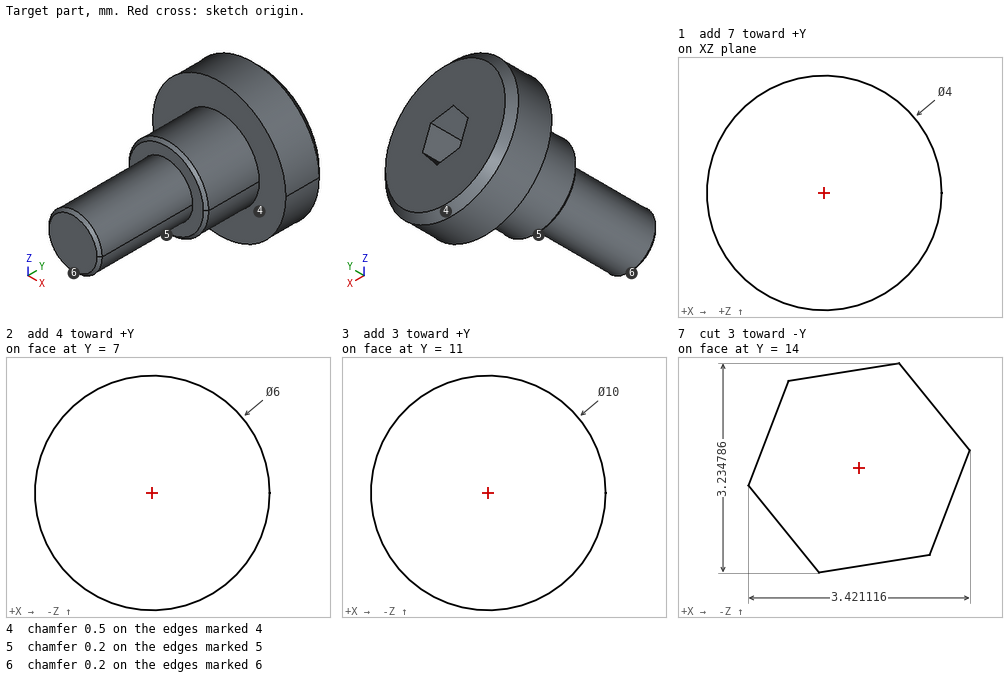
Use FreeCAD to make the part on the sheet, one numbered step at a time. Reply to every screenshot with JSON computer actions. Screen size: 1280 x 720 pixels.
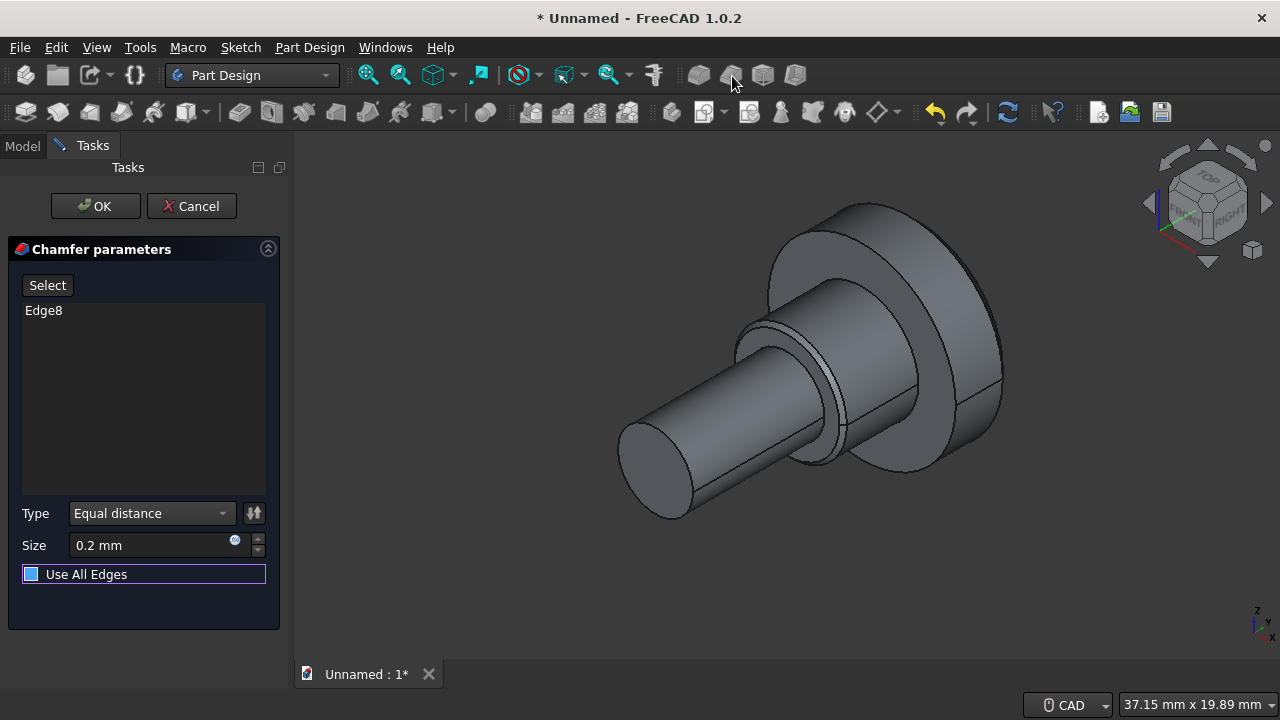
{"action": "left_click", "coordinate": [96, 206]}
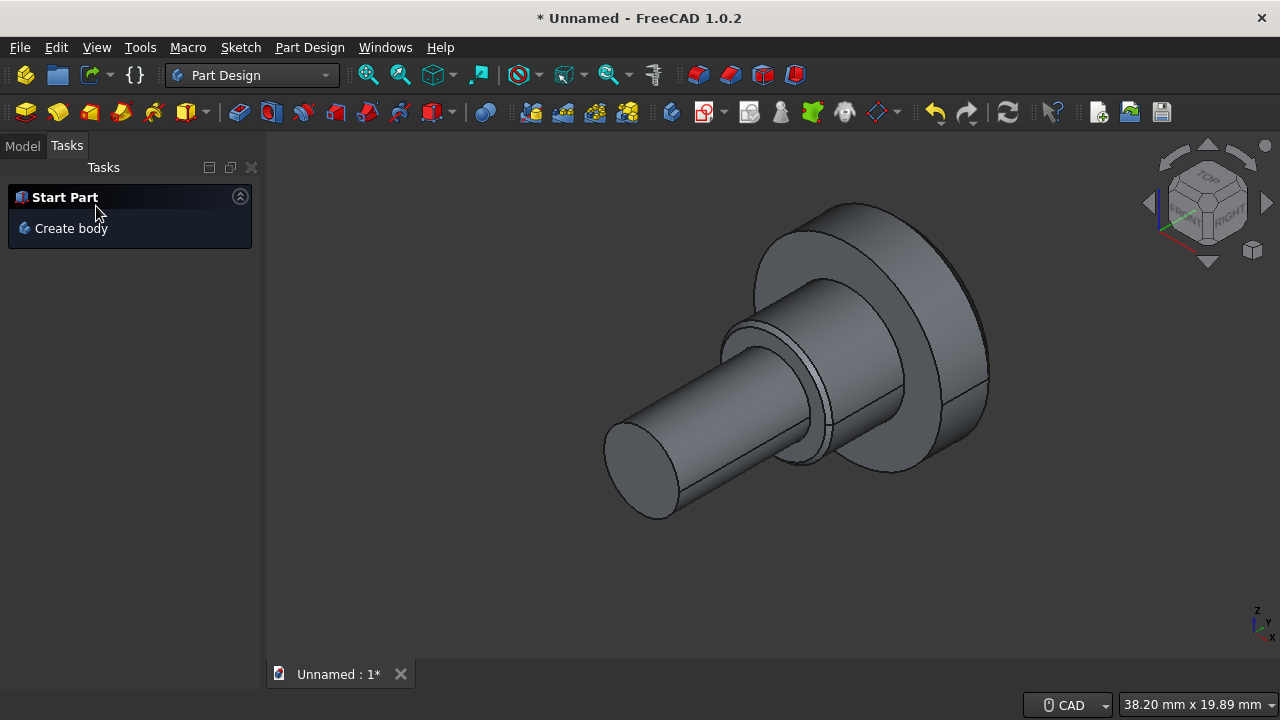
{"action": "left_click", "coordinate": [630, 422]}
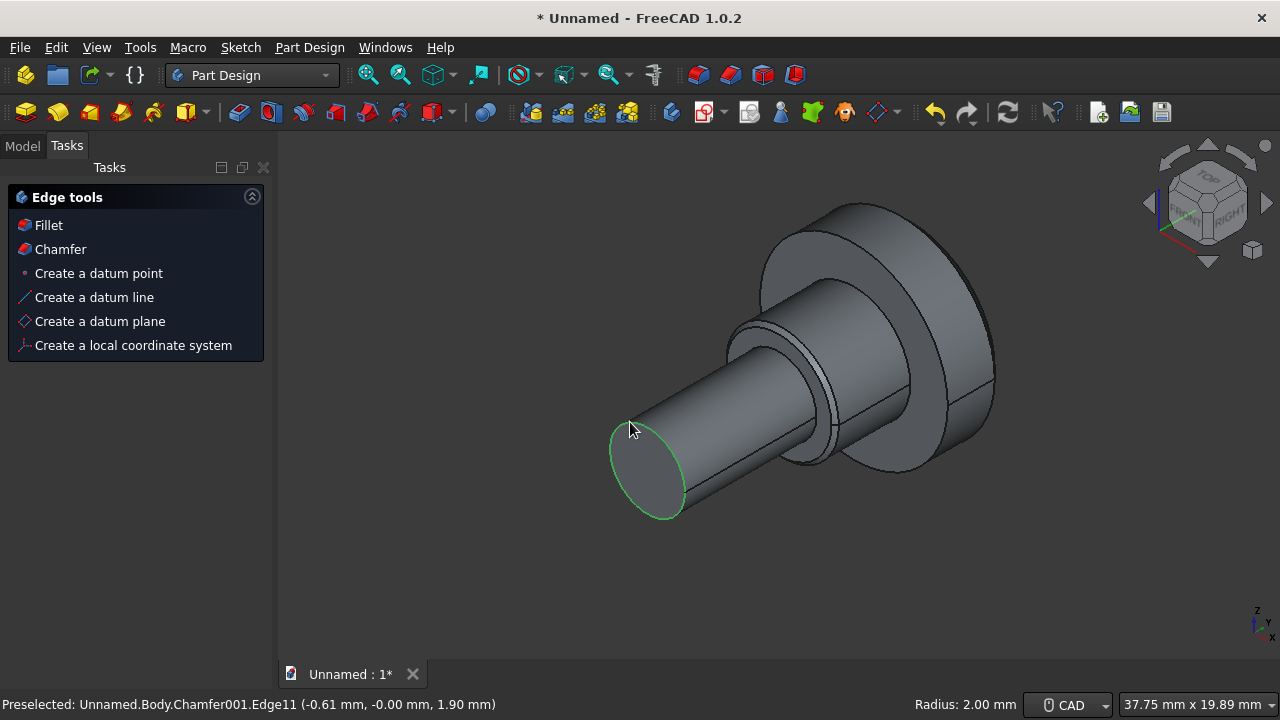
{"action": "left_click", "coordinate": [732, 76]}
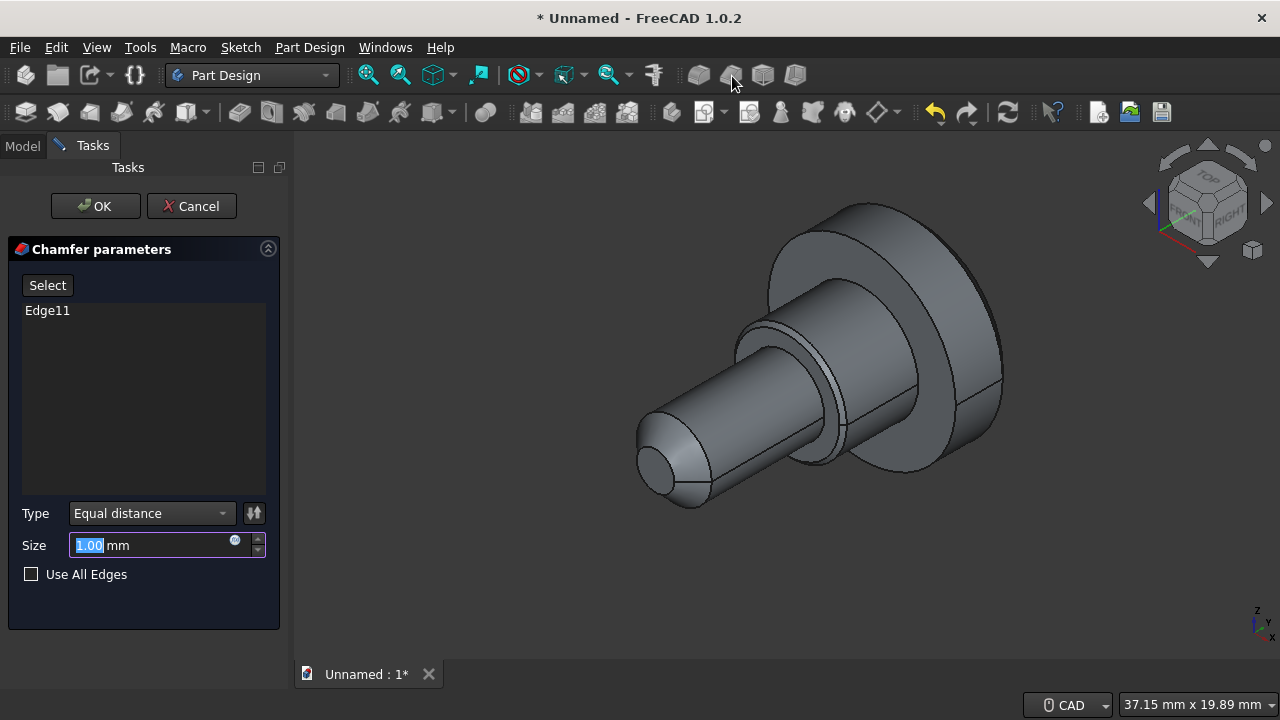
{"action": "type", "text": "0.2"}
{"action": "key", "text": "Tab"}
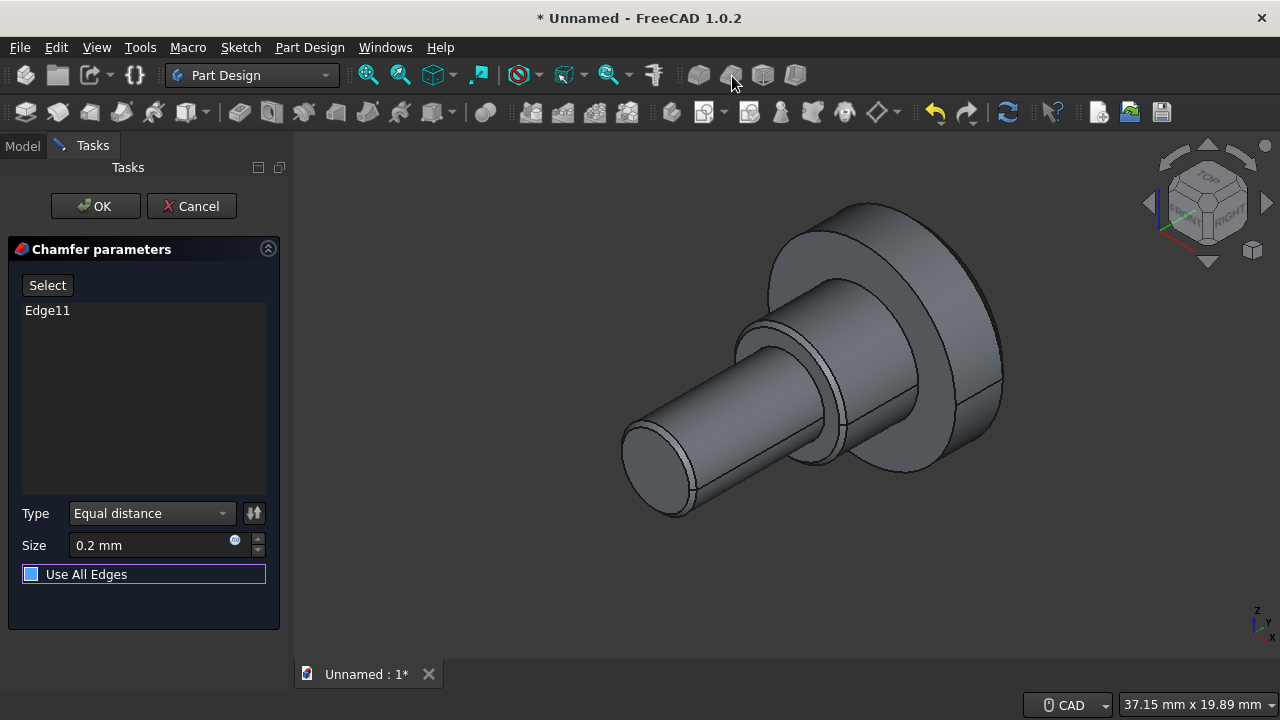
{"action": "left_click", "coordinate": [96, 206]}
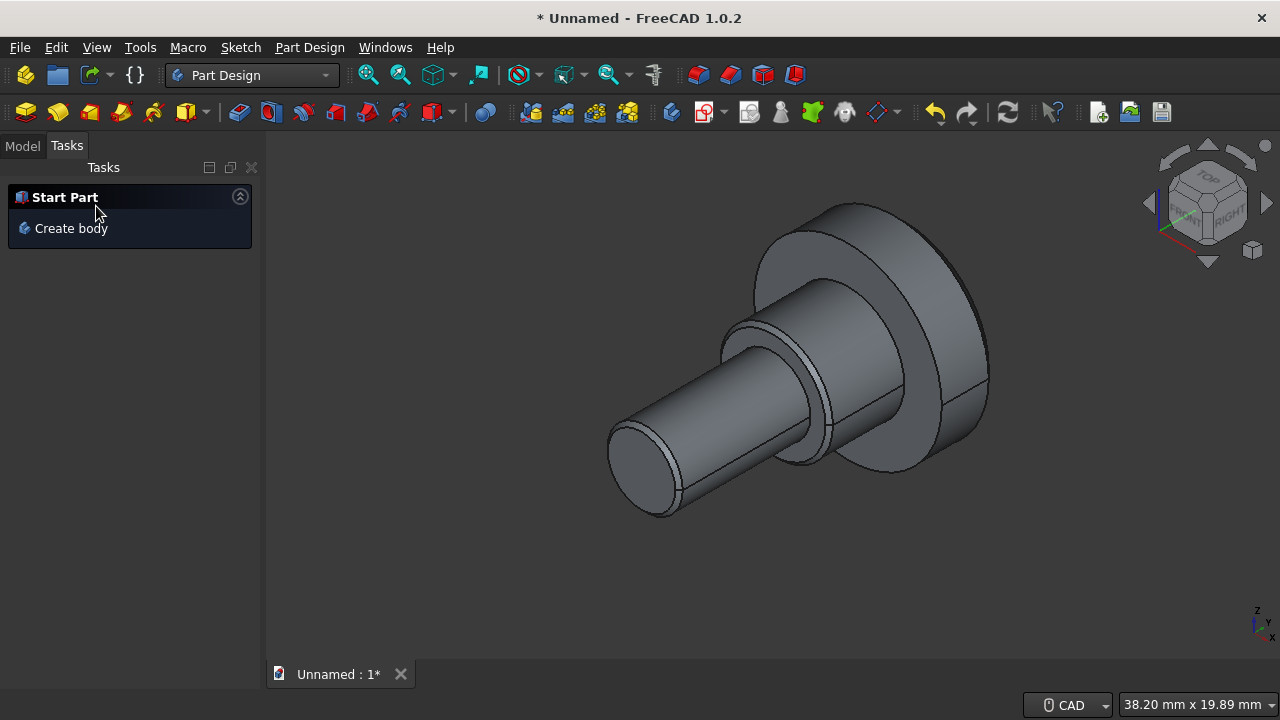
{"action": "key", "text": "4"}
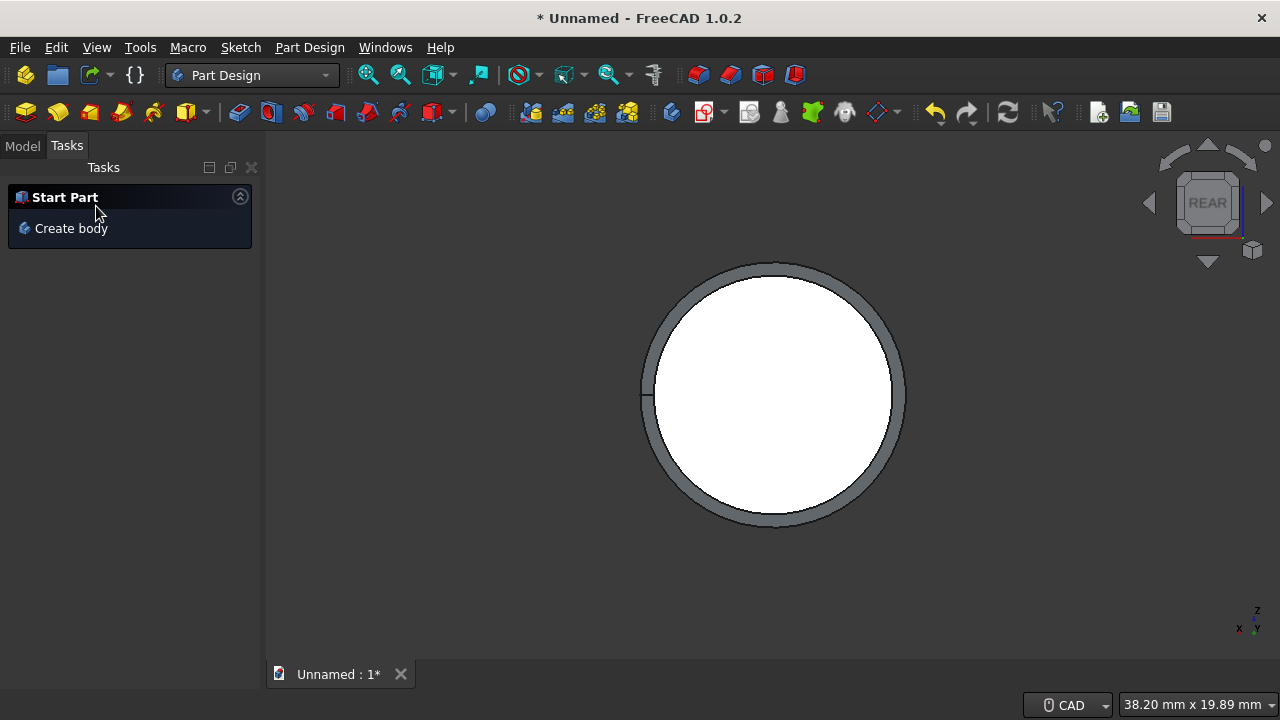
{"action": "left_click", "coordinate": [773, 394]}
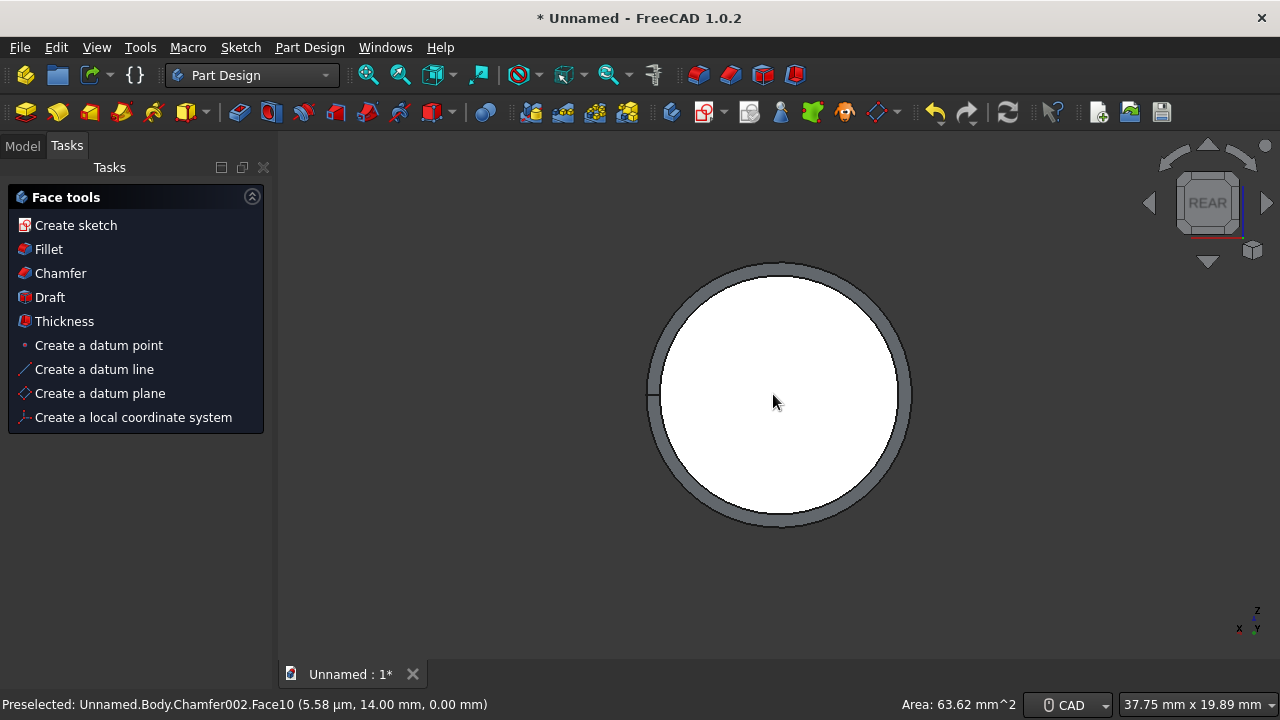
{"action": "left_click", "coordinate": [704, 112]}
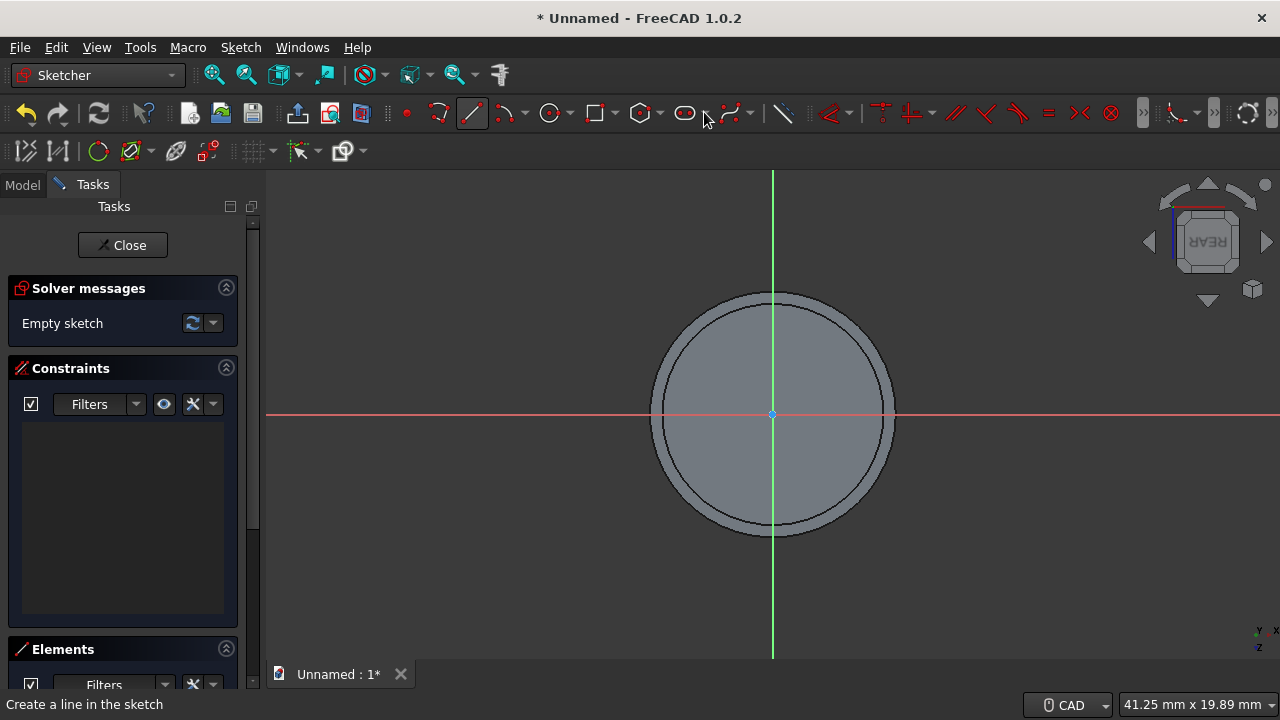
{"action": "scroll", "coordinate": [795, 415], "scroll_direction": "up", "scroll_amount": 7}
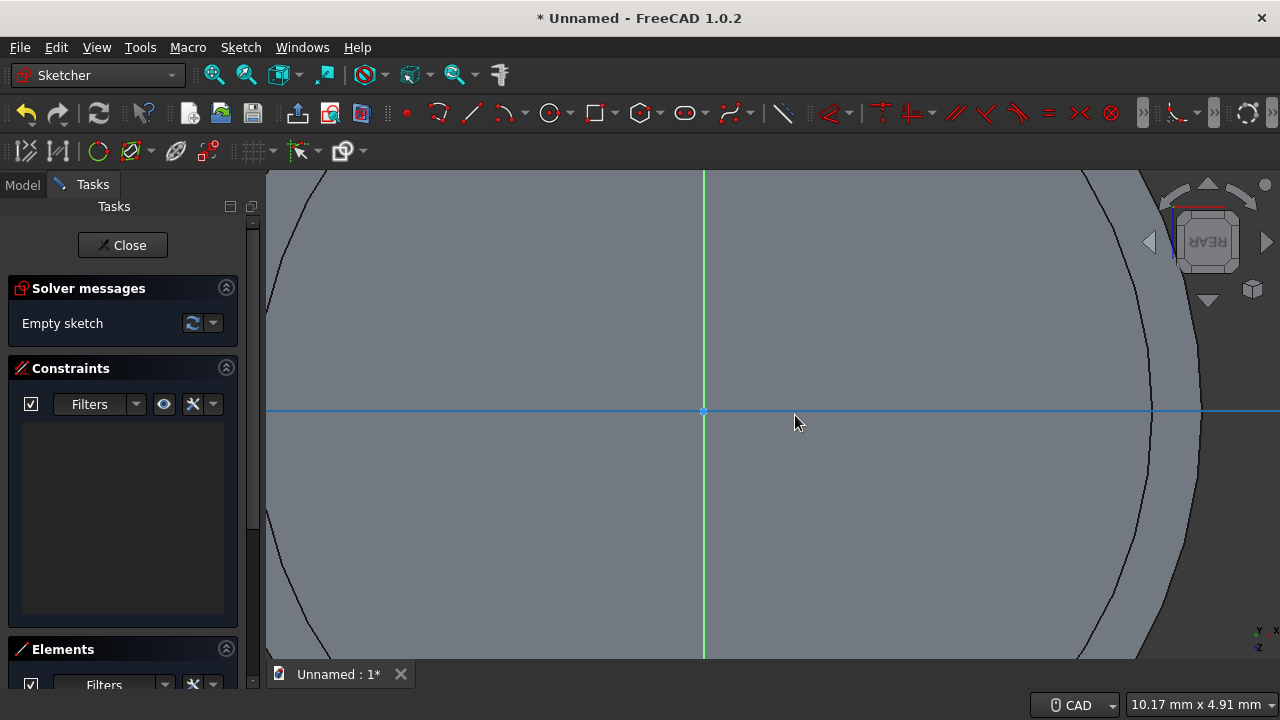
{"action": "key", "text": "g p 6"}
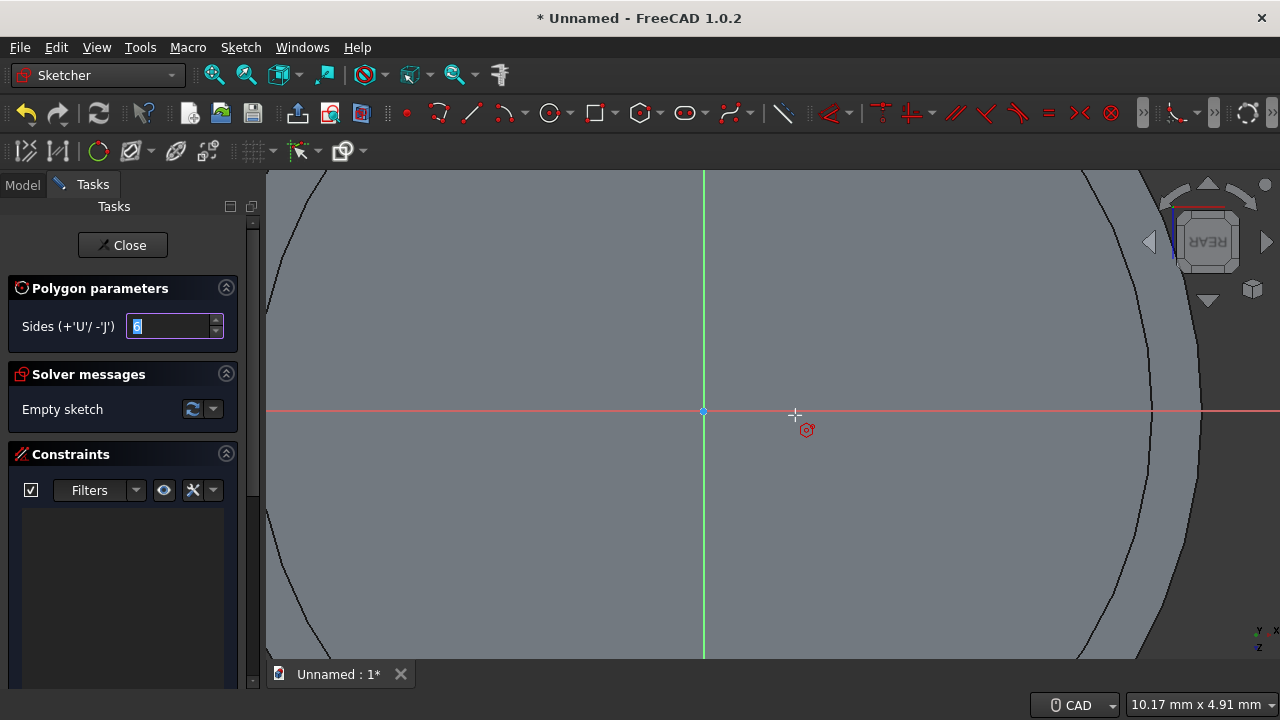
{"action": "left_click", "coordinate": [704, 411]}